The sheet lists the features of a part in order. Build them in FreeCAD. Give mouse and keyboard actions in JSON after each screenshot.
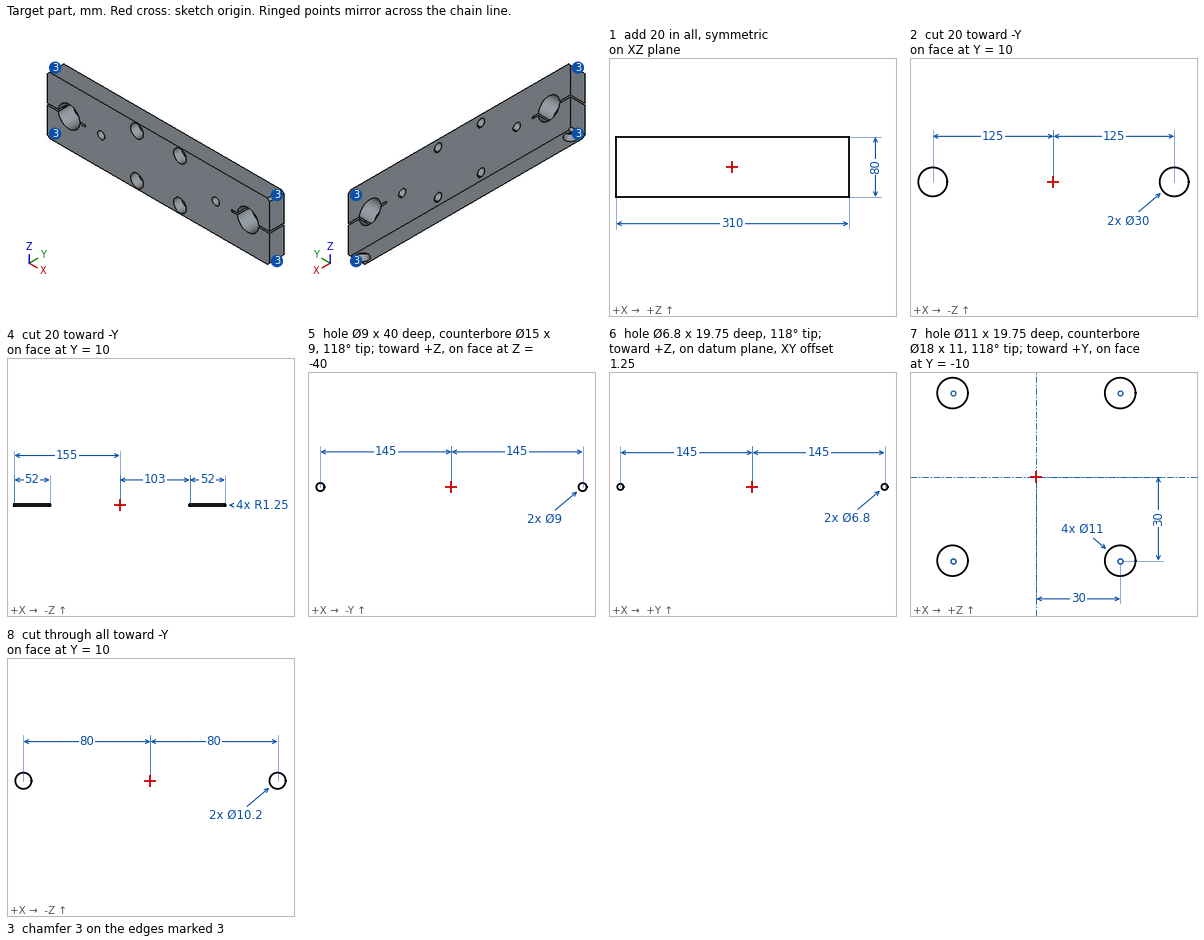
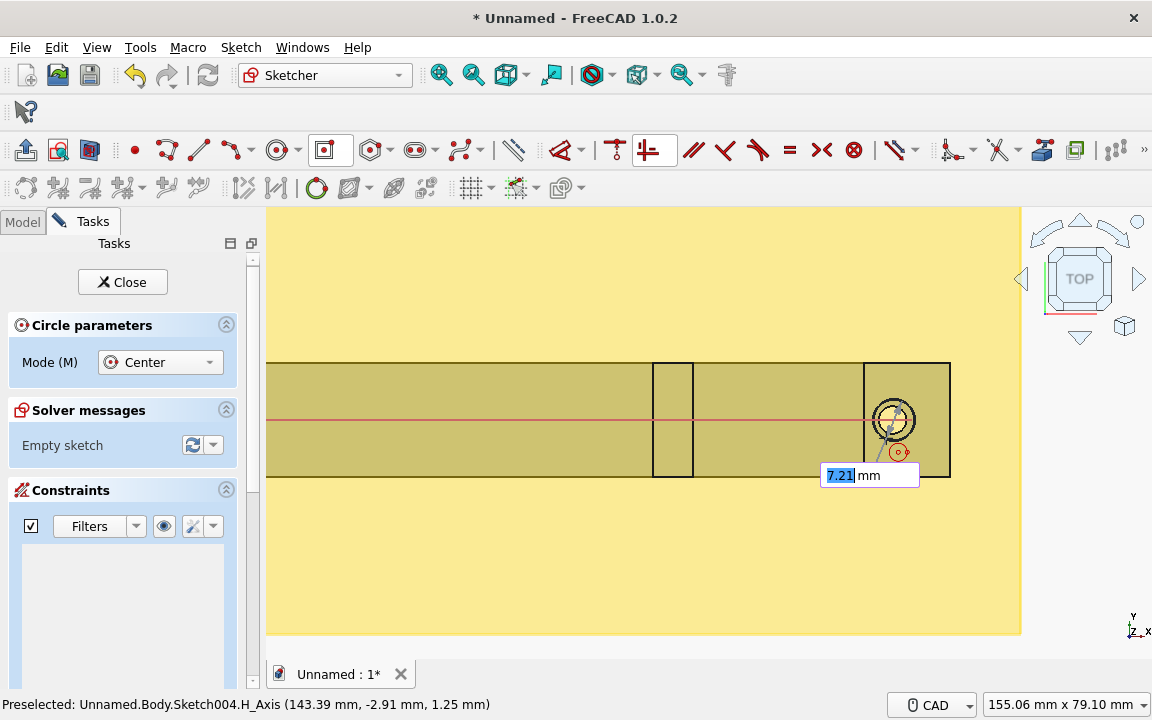
{"action": "type", "text": "6.8"}
{"action": "key", "text": "Return"}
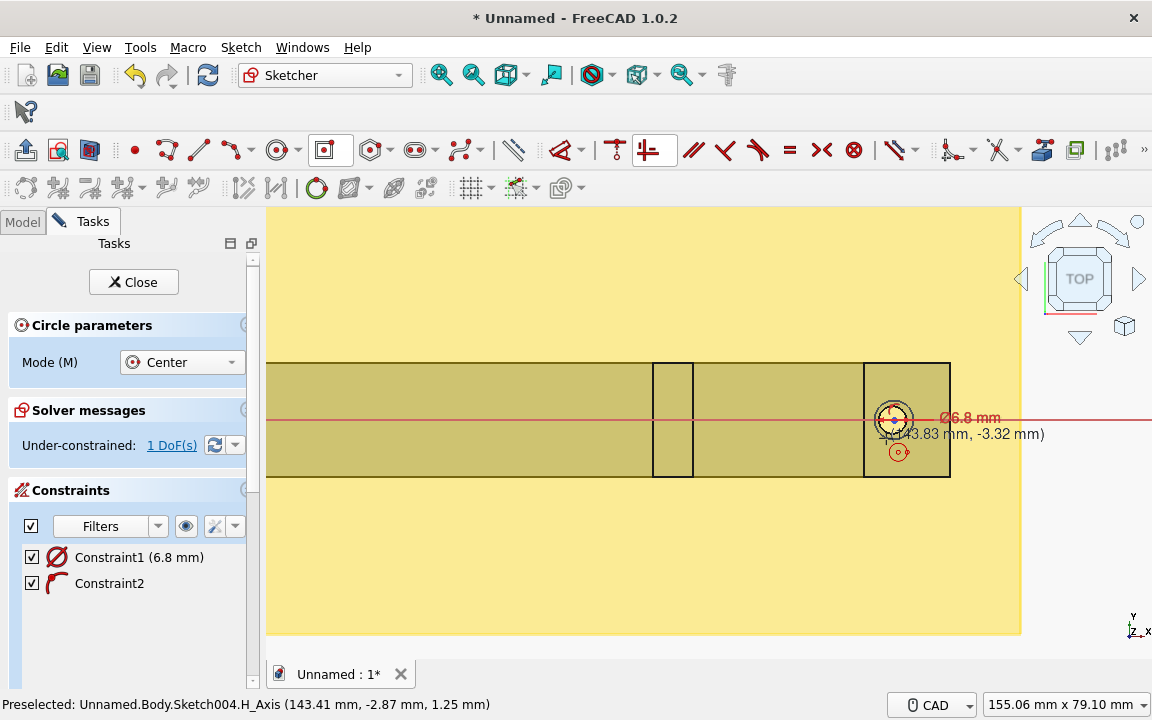
{"action": "scroll", "coordinate": [889, 439], "scroll_direction": "down", "scroll_amount": 6}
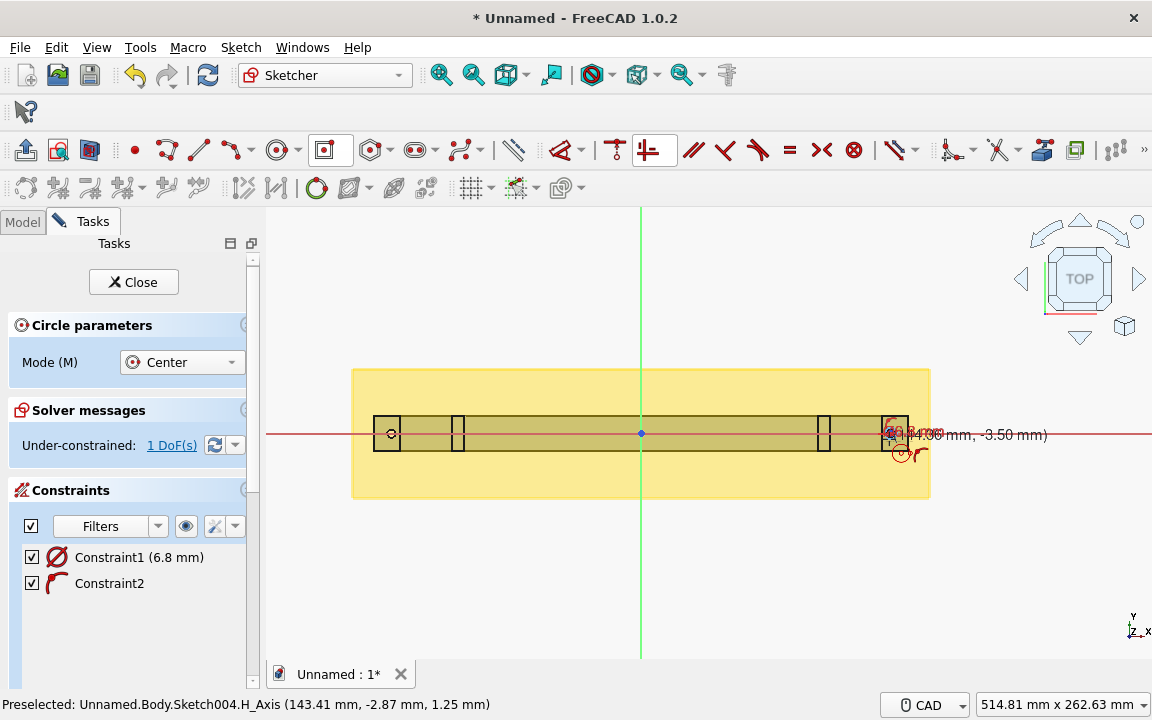
{"action": "scroll", "coordinate": [391, 434], "scroll_direction": "up", "scroll_amount": 7}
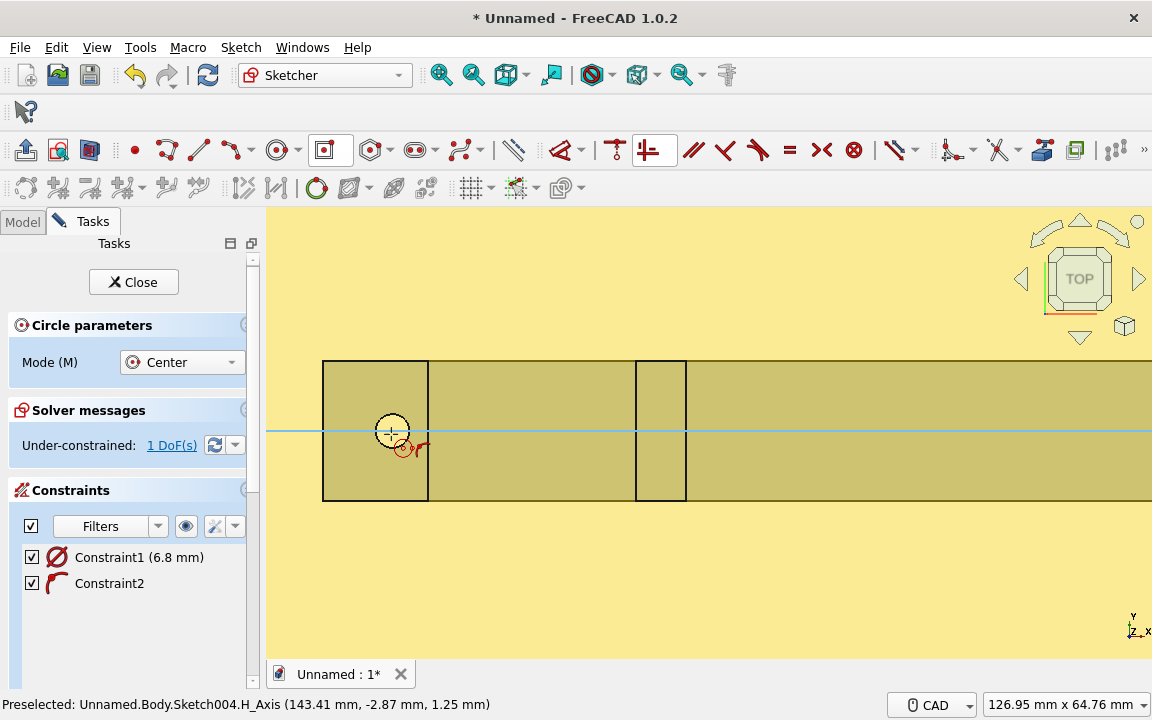
{"action": "scroll", "coordinate": [390, 434], "scroll_direction": "down", "scroll_amount": 7}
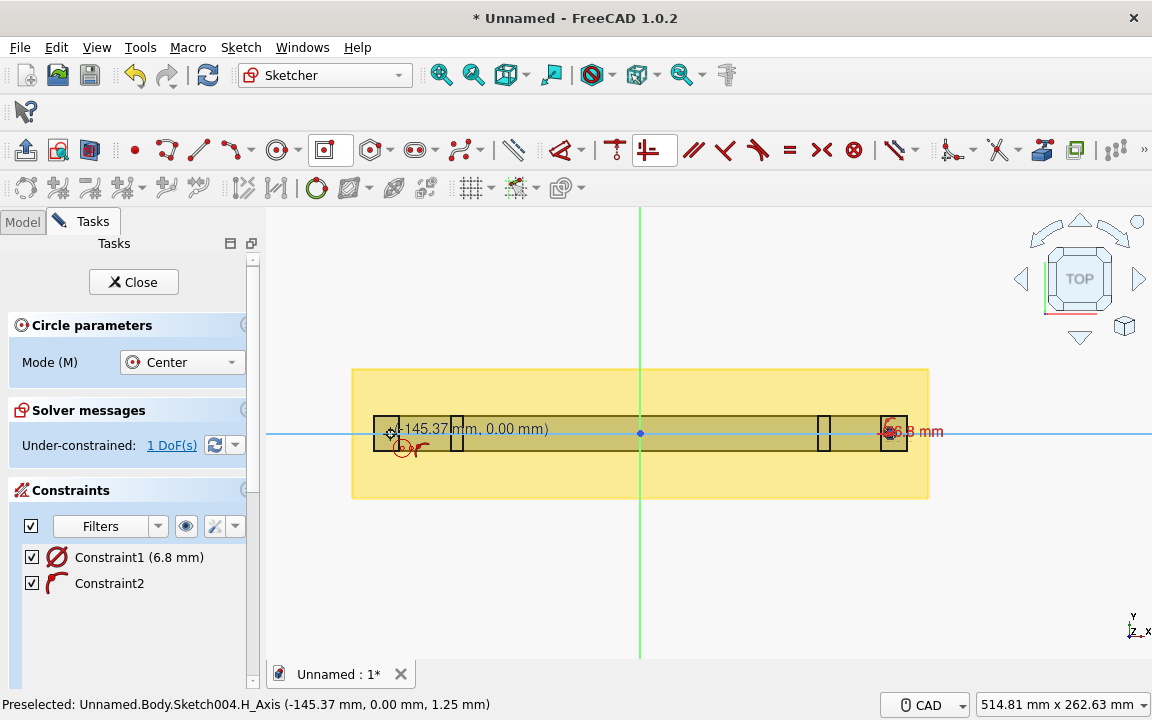
{"action": "left_click", "coordinate": [391, 434]}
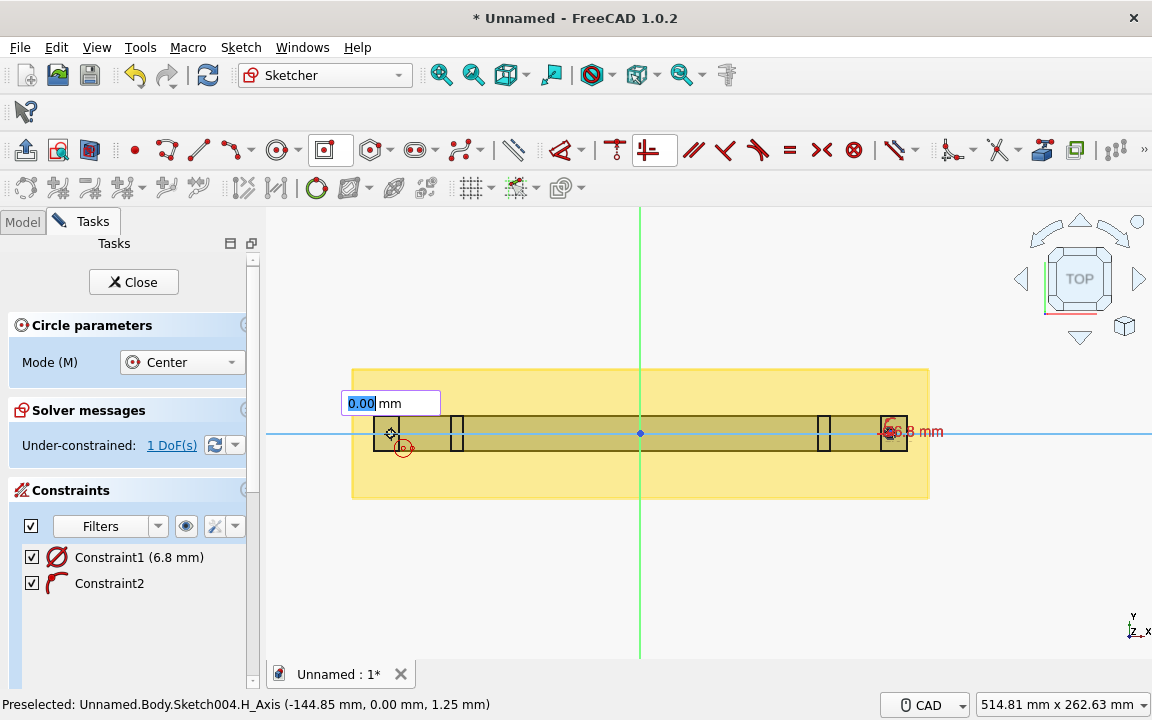
{"action": "scroll", "coordinate": [389, 439], "scroll_direction": "up", "scroll_amount": 6}
{"action": "mouse_move", "coordinate": [388, 438]}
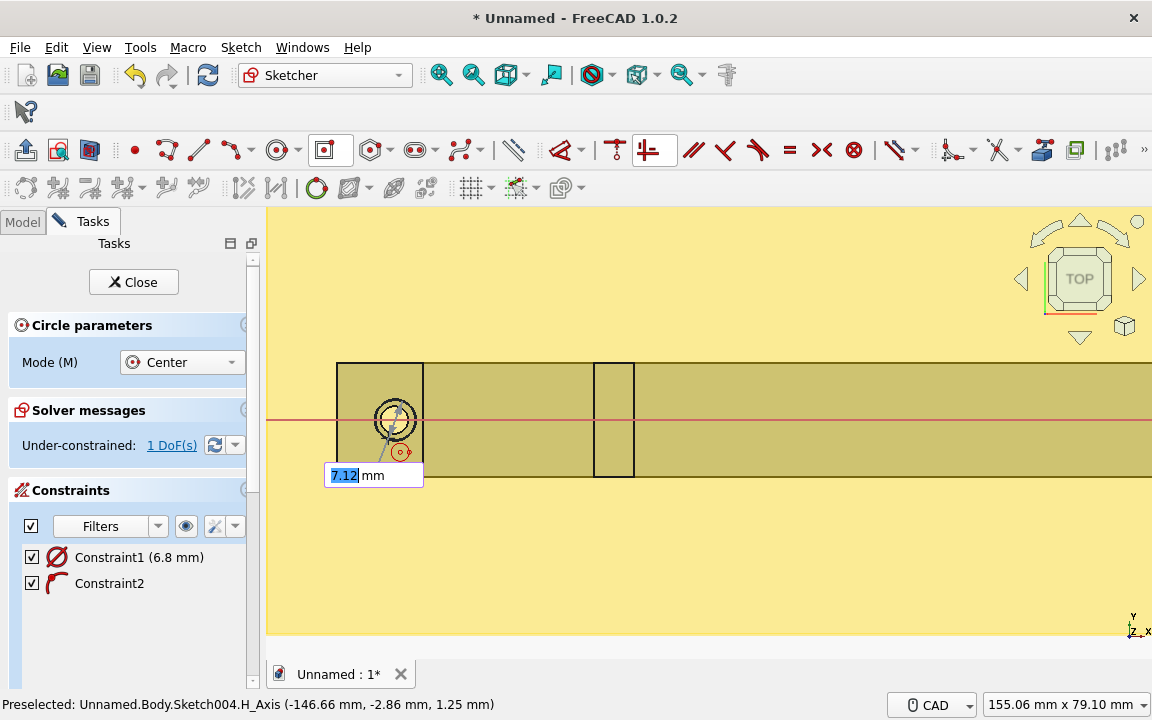
{"action": "type", "text": "6.8"}
{"action": "key", "text": "Return"}
{"action": "key", "text": "Escape"}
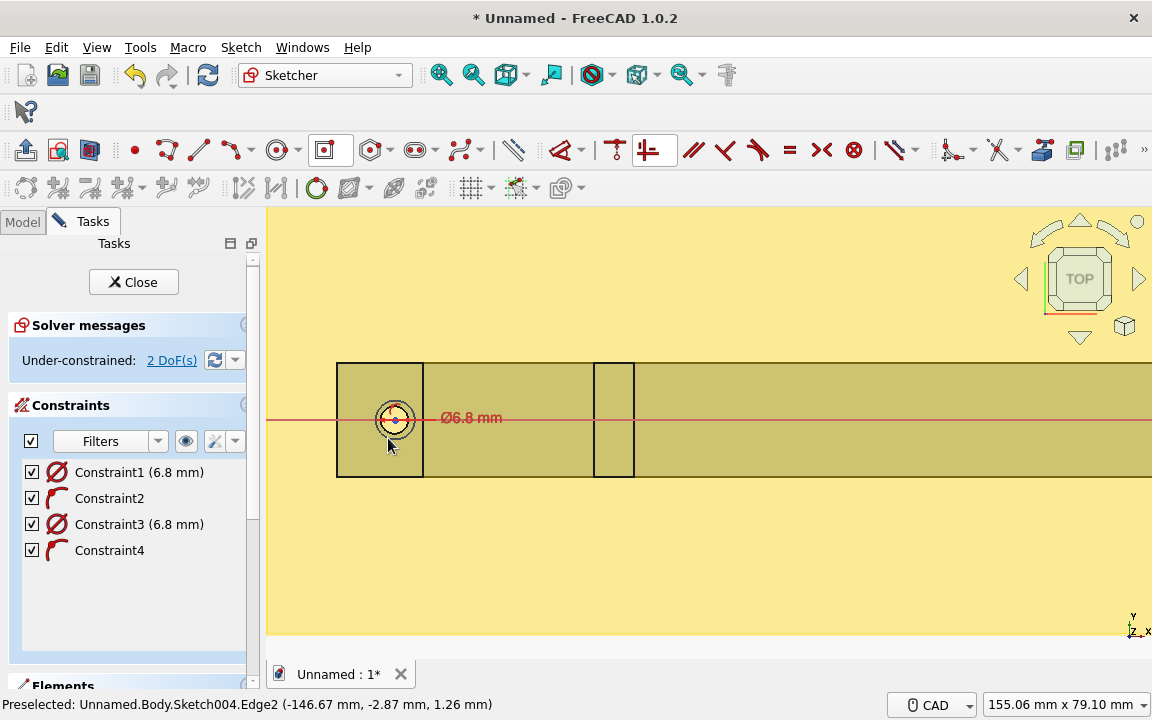
{"action": "left_click", "coordinate": [560, 150]}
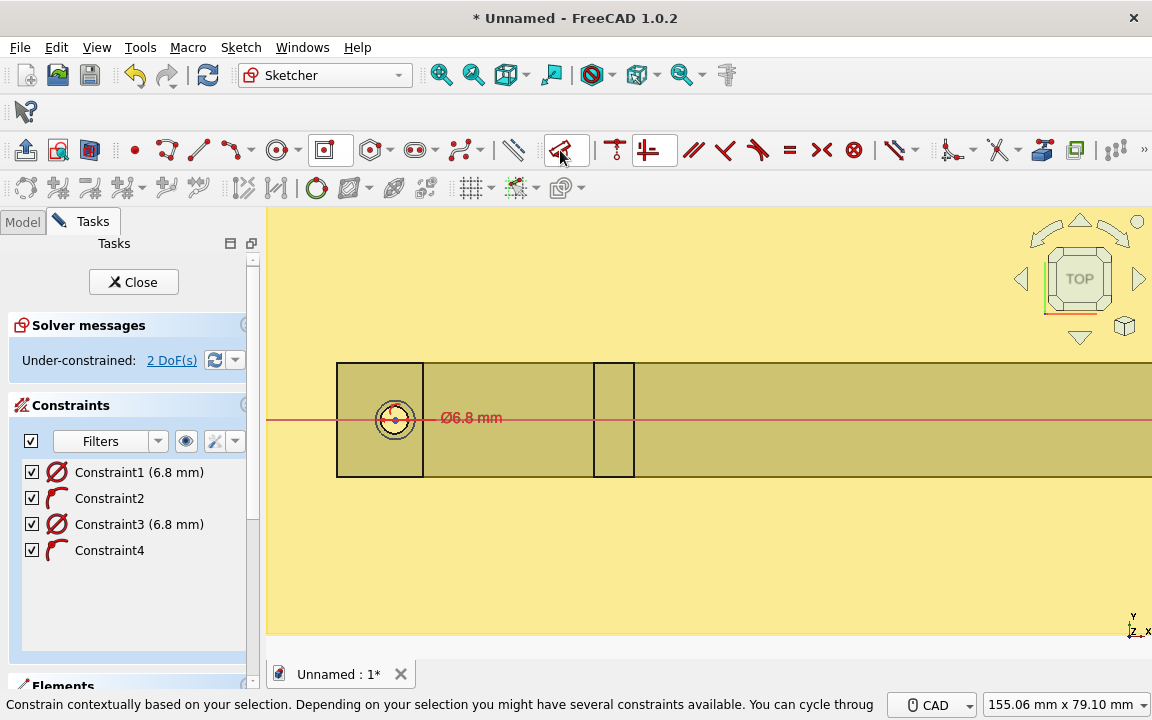
{"action": "scroll", "coordinate": [389, 439], "scroll_direction": "down", "scroll_amount": 6}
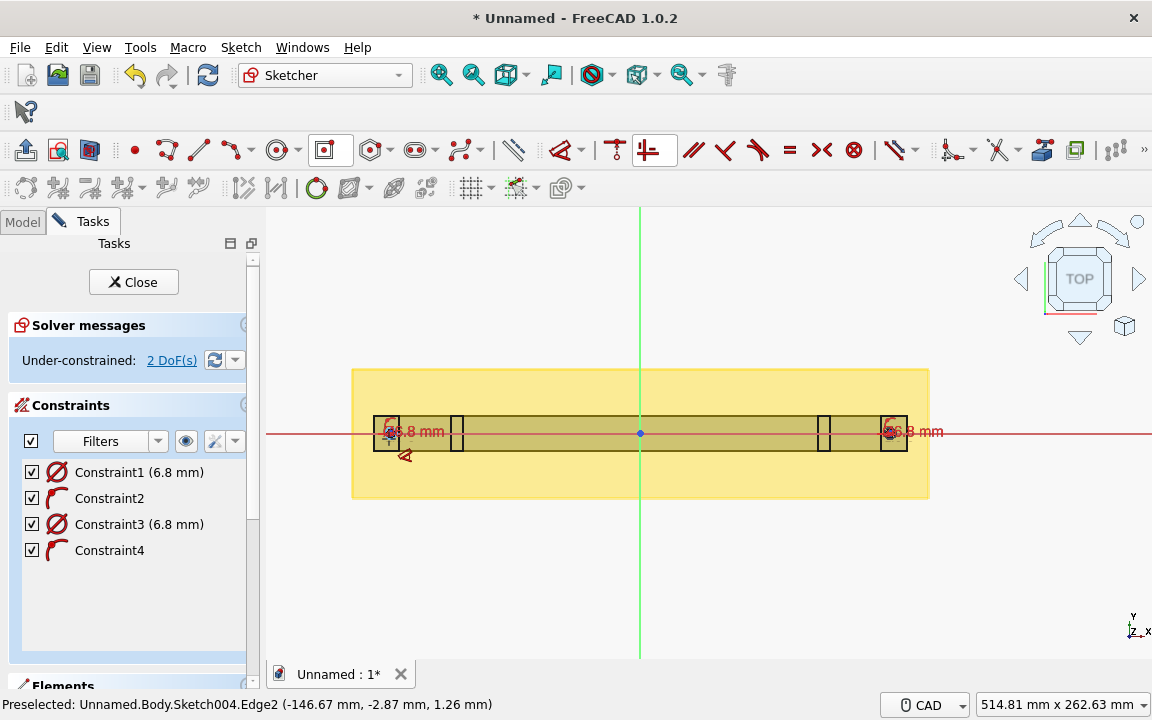
{"action": "left_click", "coordinate": [890, 434]}
{"action": "left_click", "coordinate": [765, 468]}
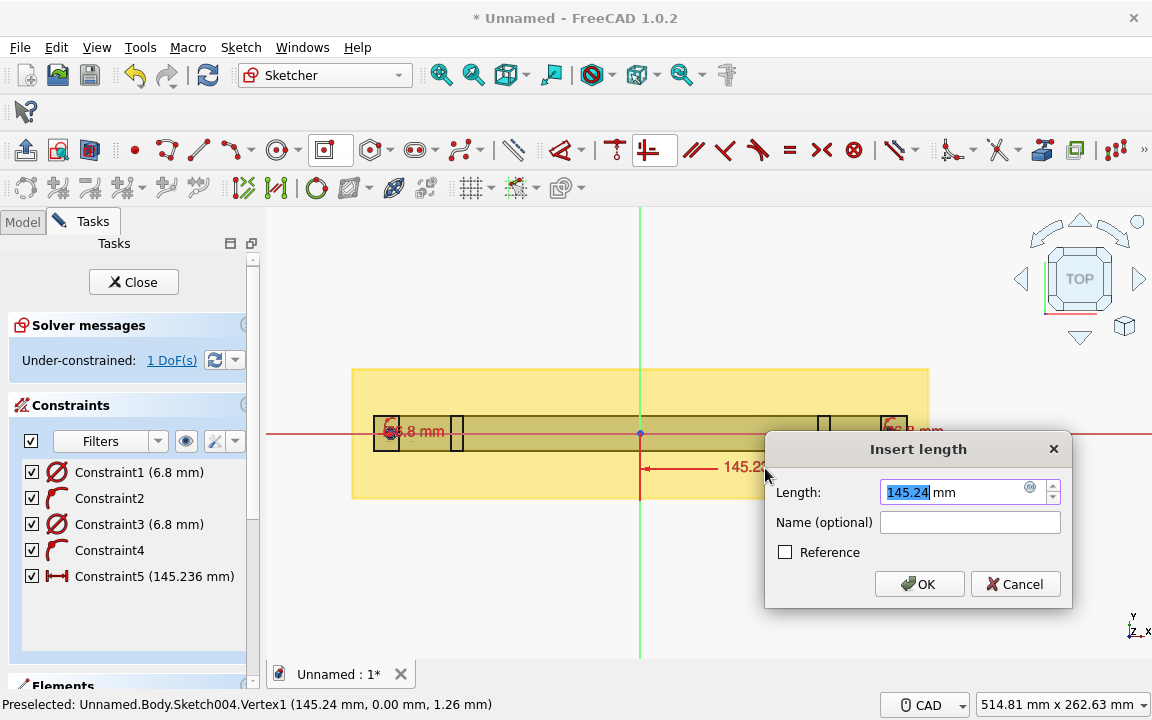
{"action": "type", "text": "145"}
{"action": "key", "text": "Return"}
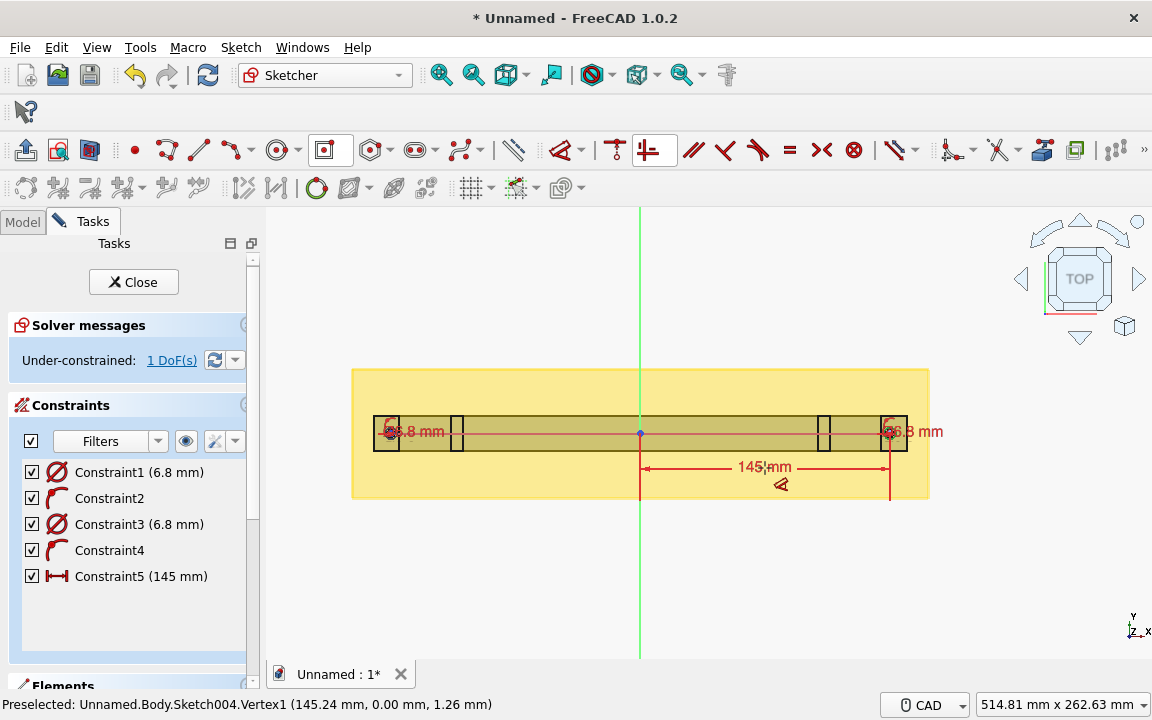
{"action": "left_click", "coordinate": [391, 434]}
{"action": "left_click", "coordinate": [516, 468]}